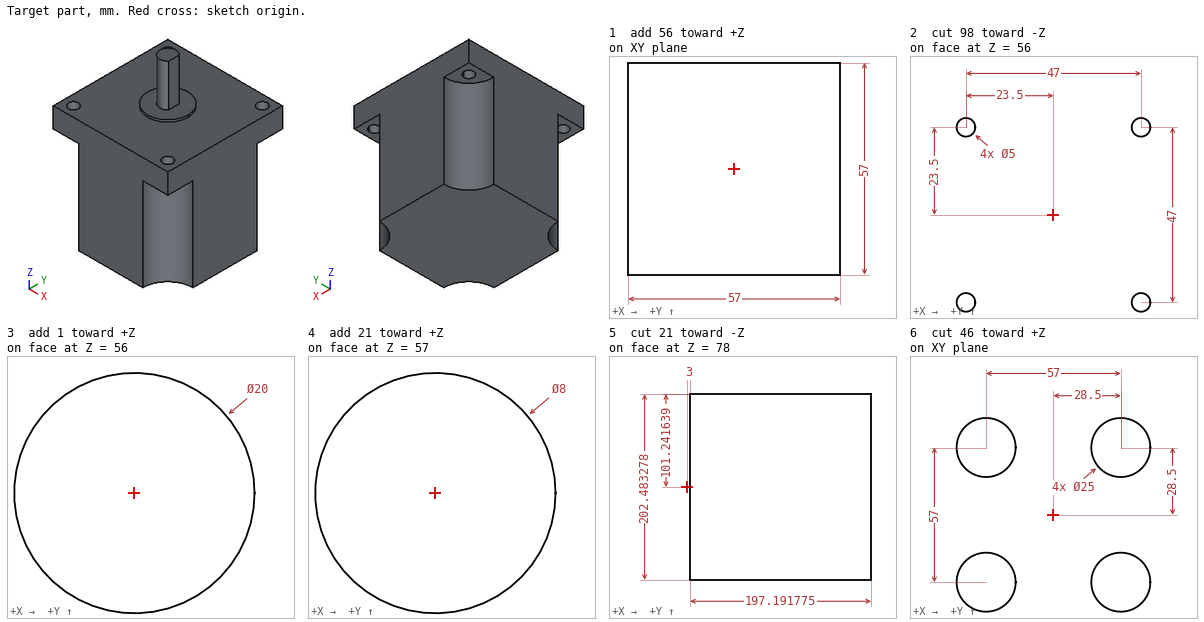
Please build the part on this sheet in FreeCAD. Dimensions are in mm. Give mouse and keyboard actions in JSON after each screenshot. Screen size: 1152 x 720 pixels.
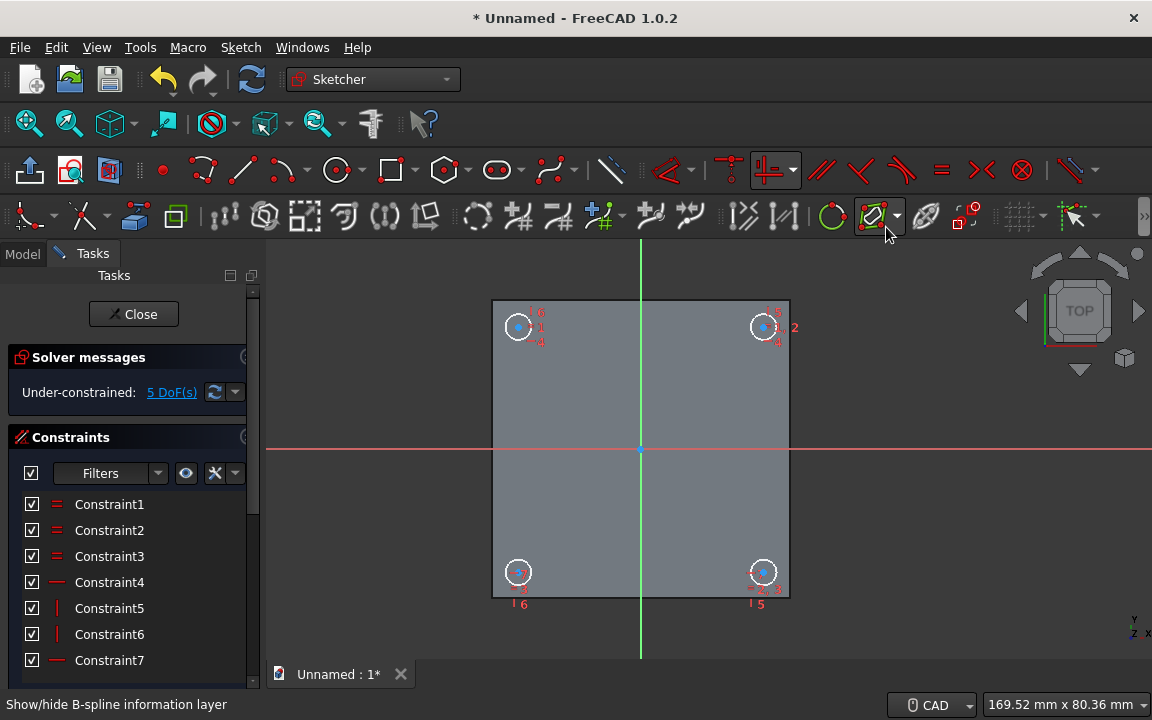
{"action": "left_click", "coordinate": [666, 170]}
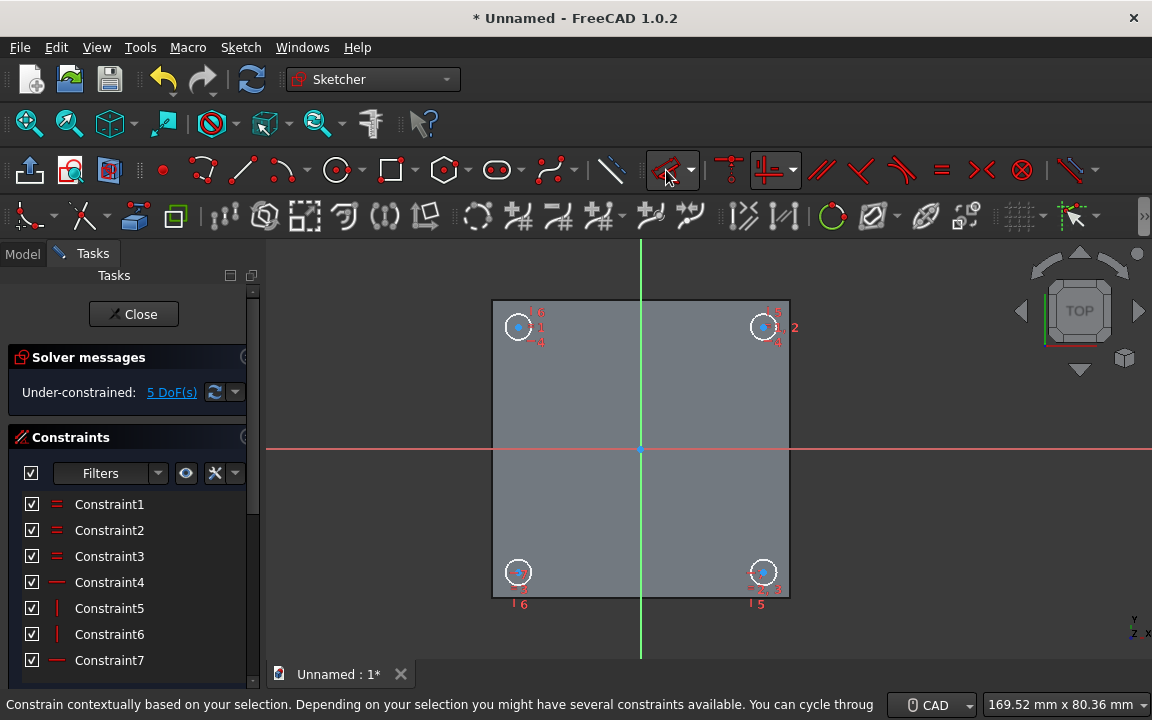
{"action": "scroll", "coordinate": [527, 318], "scroll_direction": "up", "scroll_amount": 3}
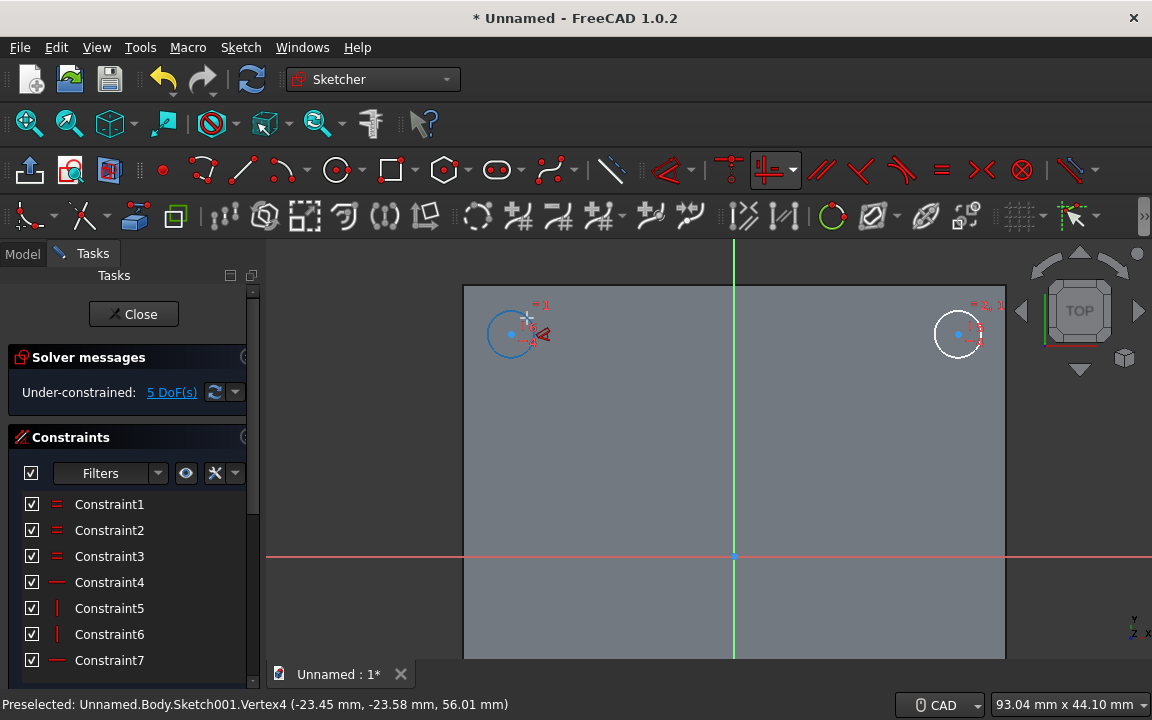
{"action": "left_click", "coordinate": [528, 318]}
{"action": "left_click", "coordinate": [551, 296]}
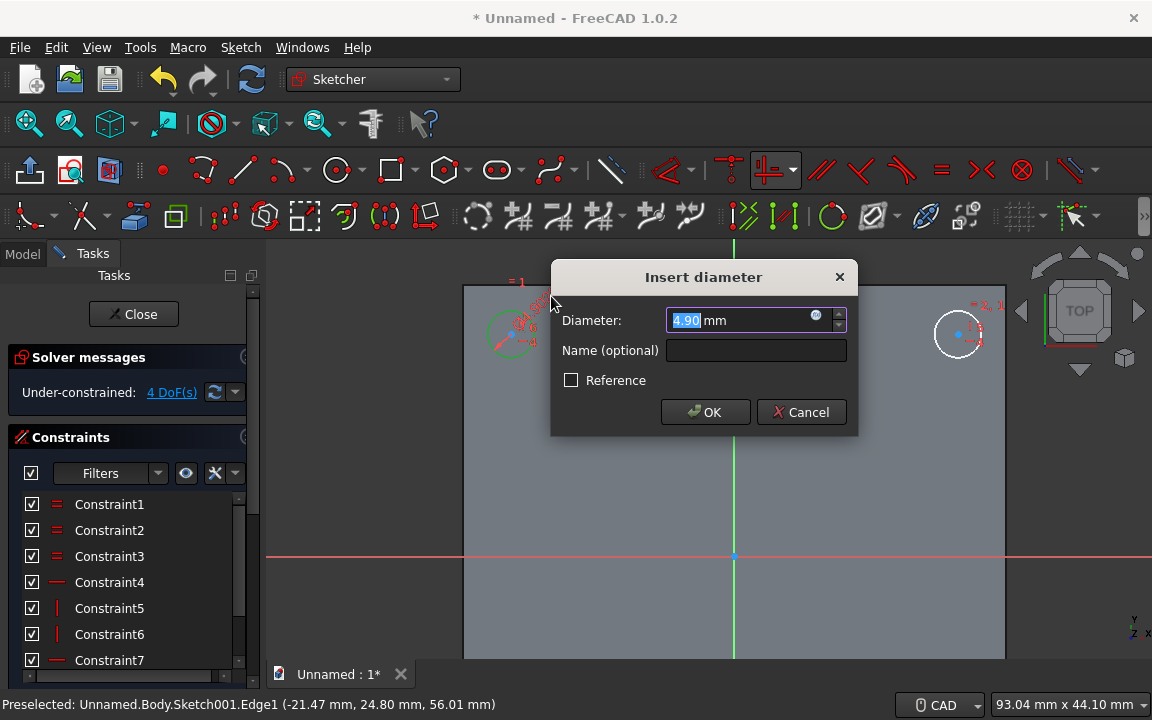
{"action": "type", "text": "5"}
{"action": "key", "text": "Return"}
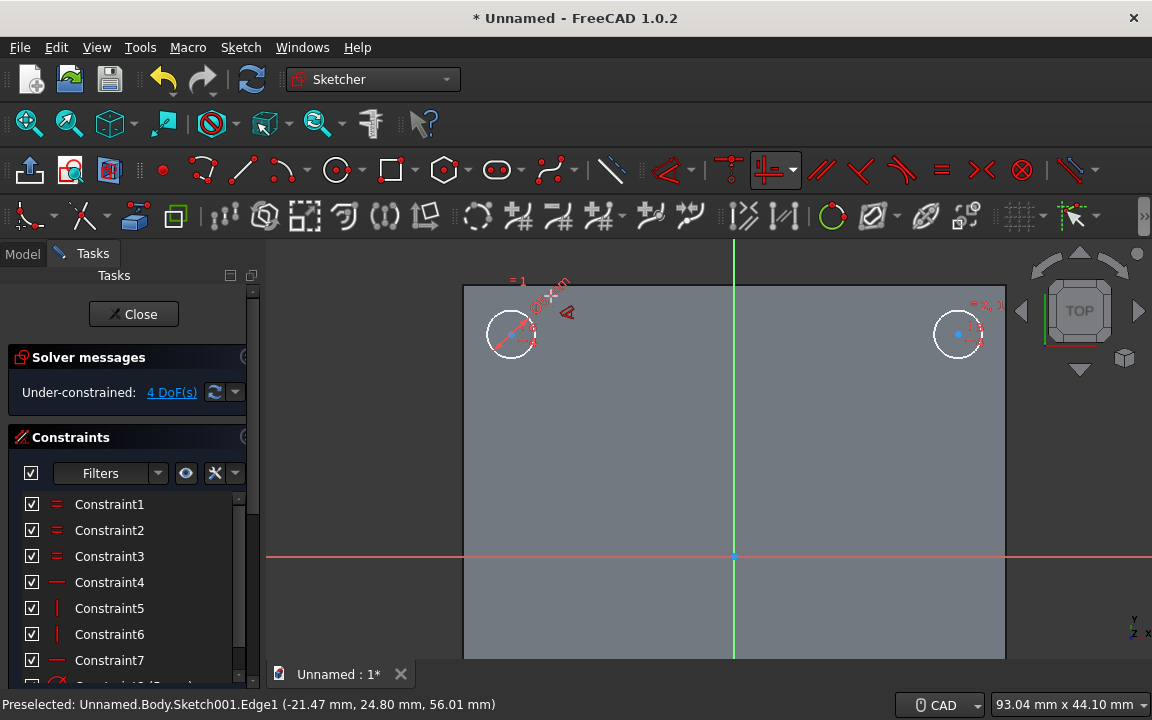
{"action": "left_click", "coordinate": [511, 334]}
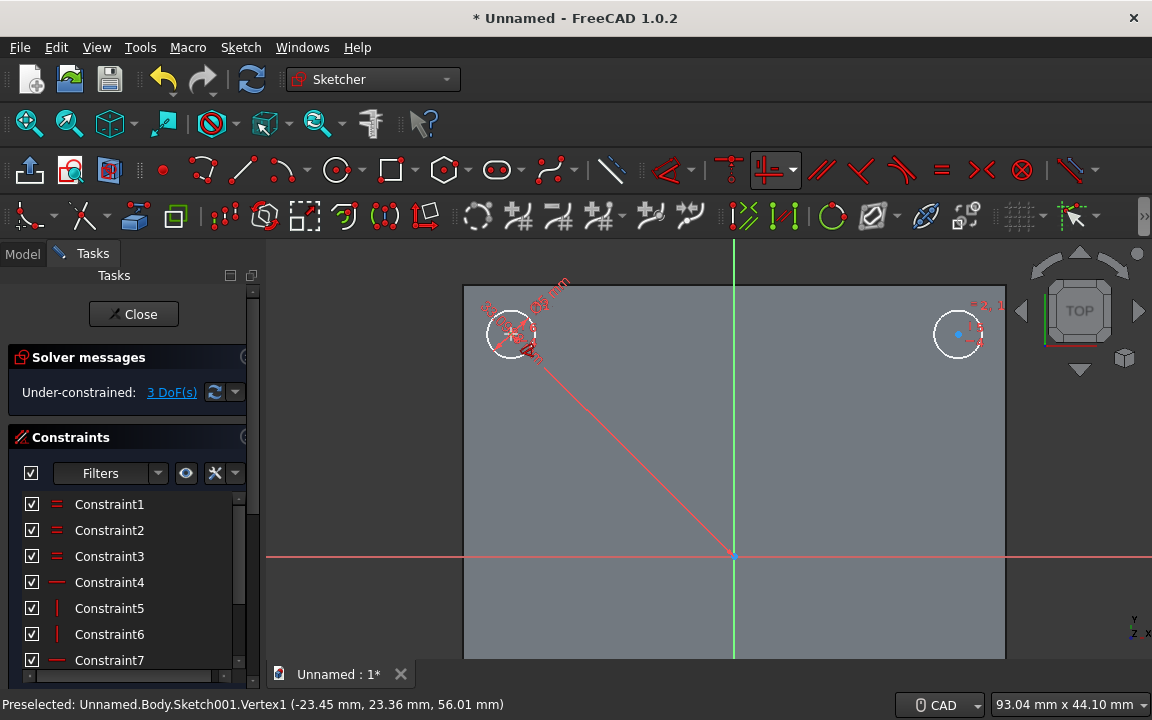
{"action": "left_click", "coordinate": [958, 334]}
{"action": "left_click", "coordinate": [632, 300]}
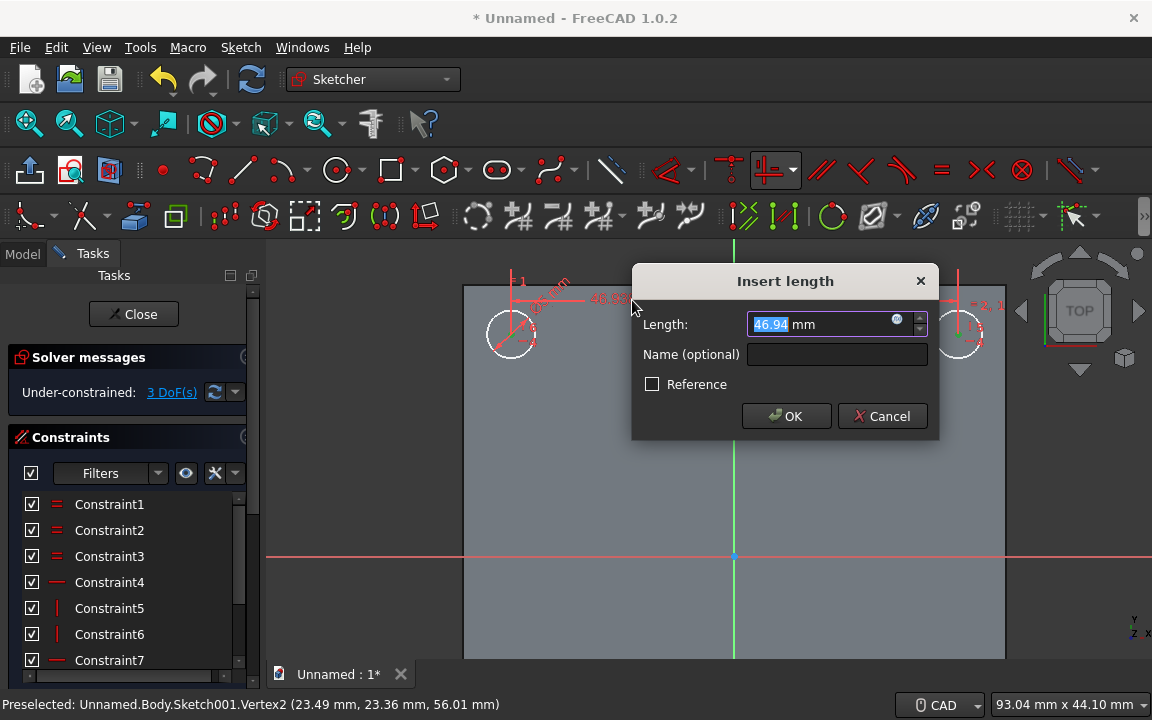
{"action": "type", "text": "47"}
{"action": "key", "text": "Return"}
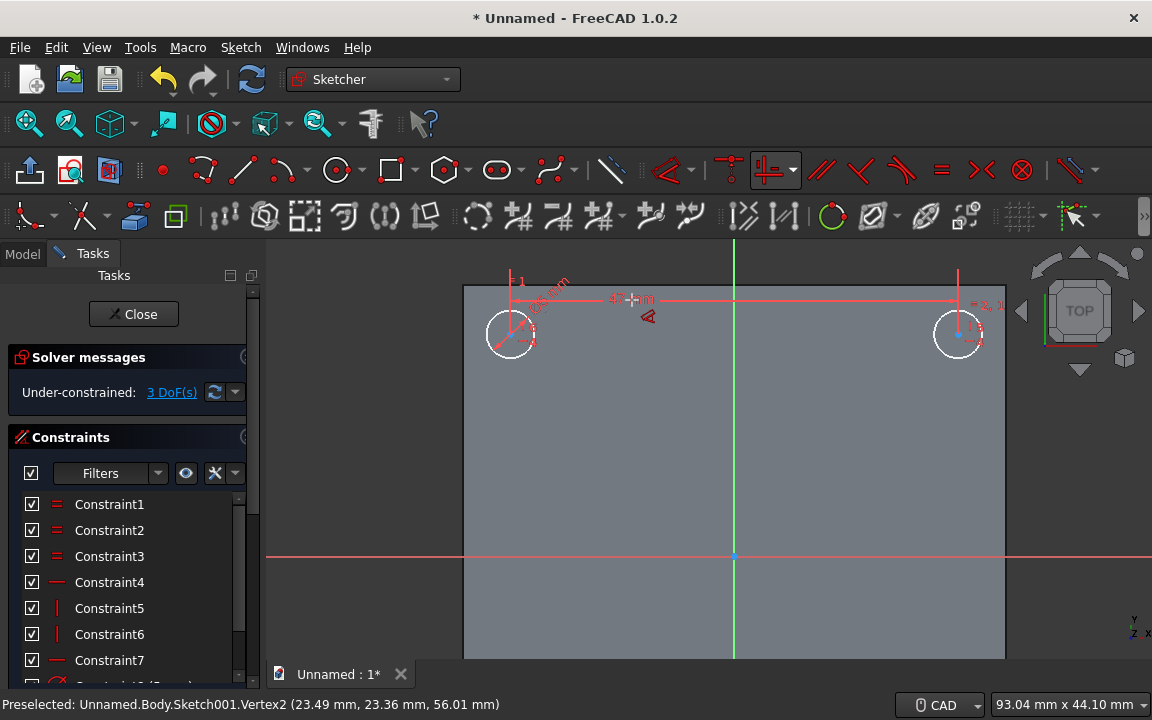
{"action": "left_click", "coordinate": [958, 334]}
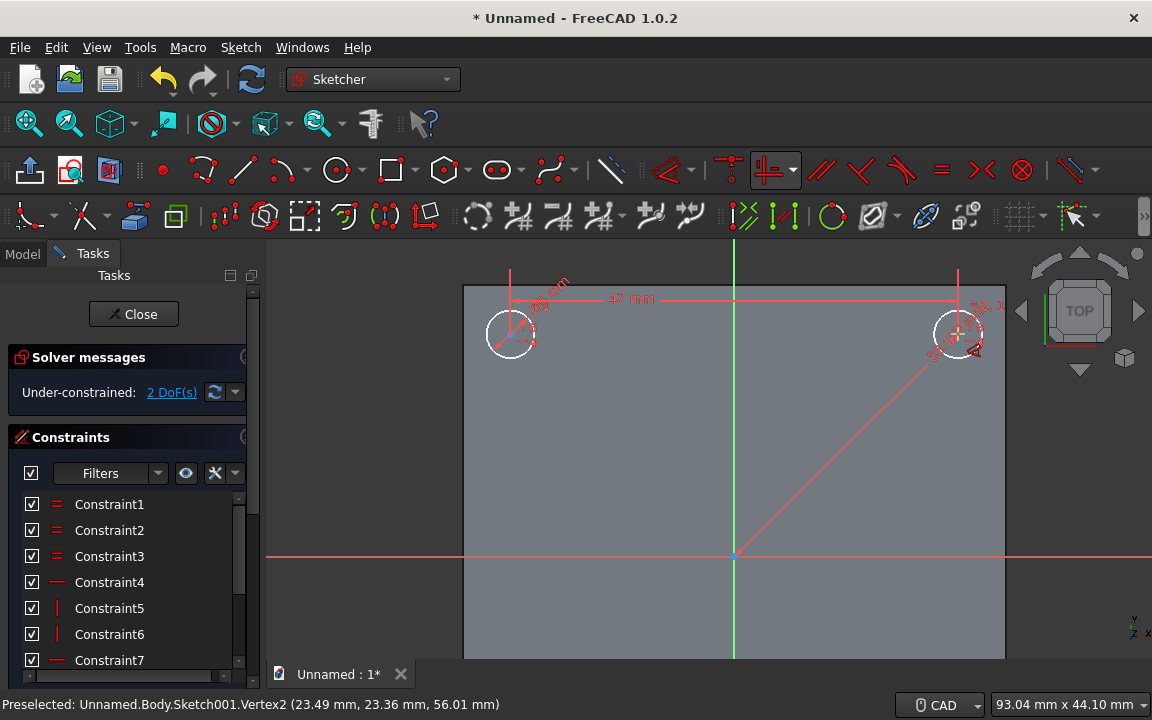
{"action": "scroll", "coordinate": [526, 318], "scroll_direction": "down", "scroll_amount": 3}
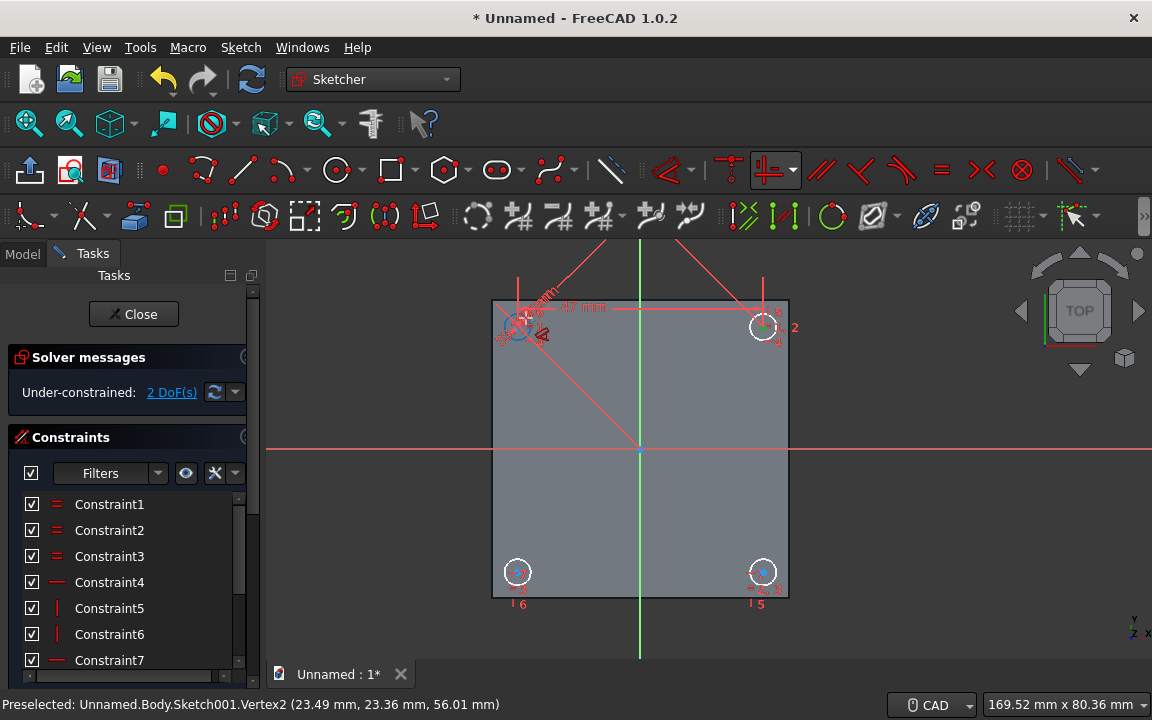
{"action": "left_click", "coordinate": [763, 572]}
{"action": "left_click", "coordinate": [797, 393]}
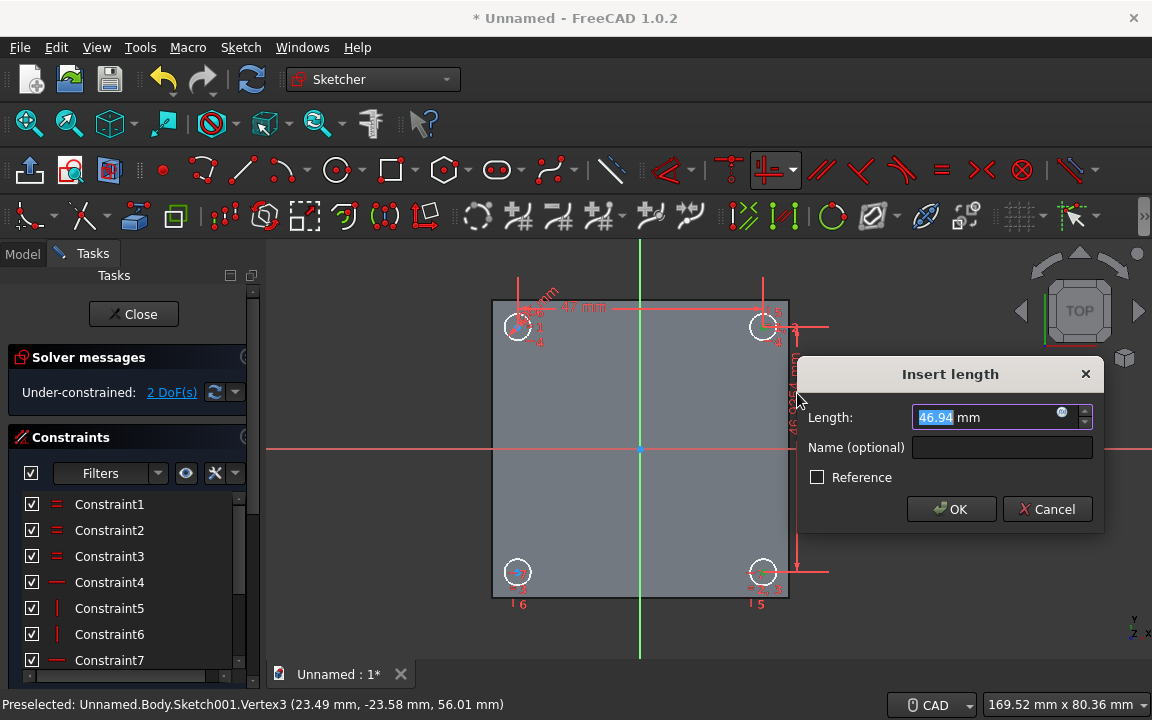
{"action": "type", "text": "47"}
{"action": "key", "text": "Return"}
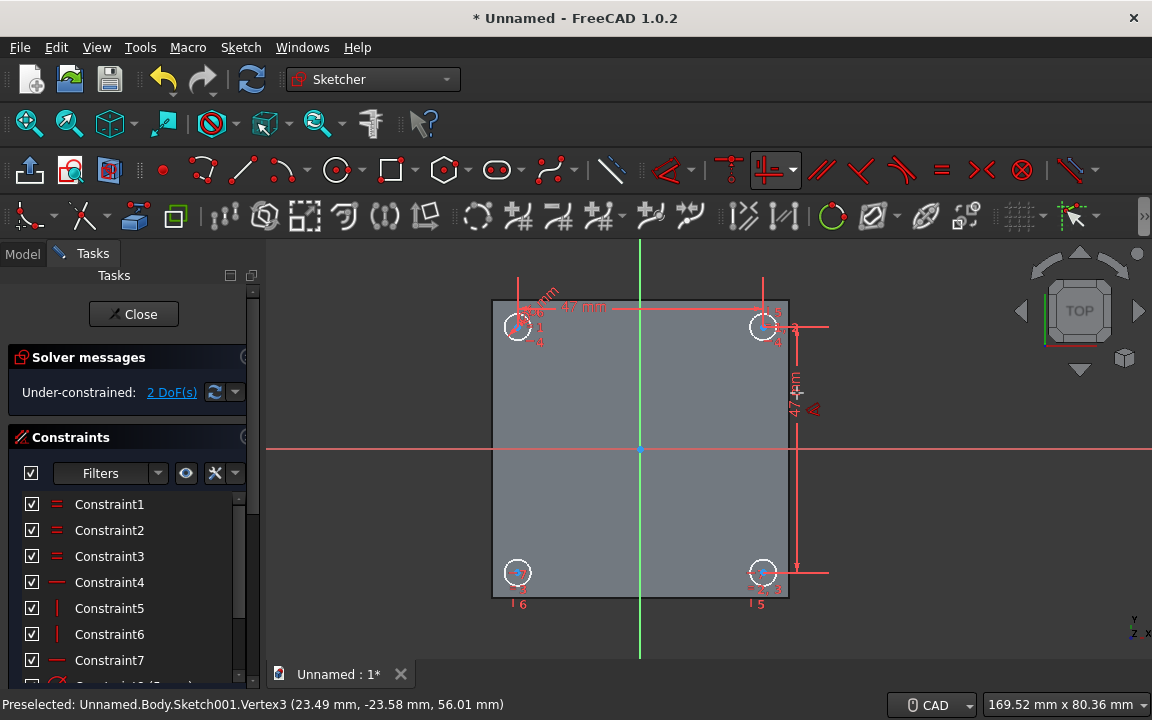
{"action": "left_click", "coordinate": [518, 327]}
{"action": "left_click", "coordinate": [579, 483]}